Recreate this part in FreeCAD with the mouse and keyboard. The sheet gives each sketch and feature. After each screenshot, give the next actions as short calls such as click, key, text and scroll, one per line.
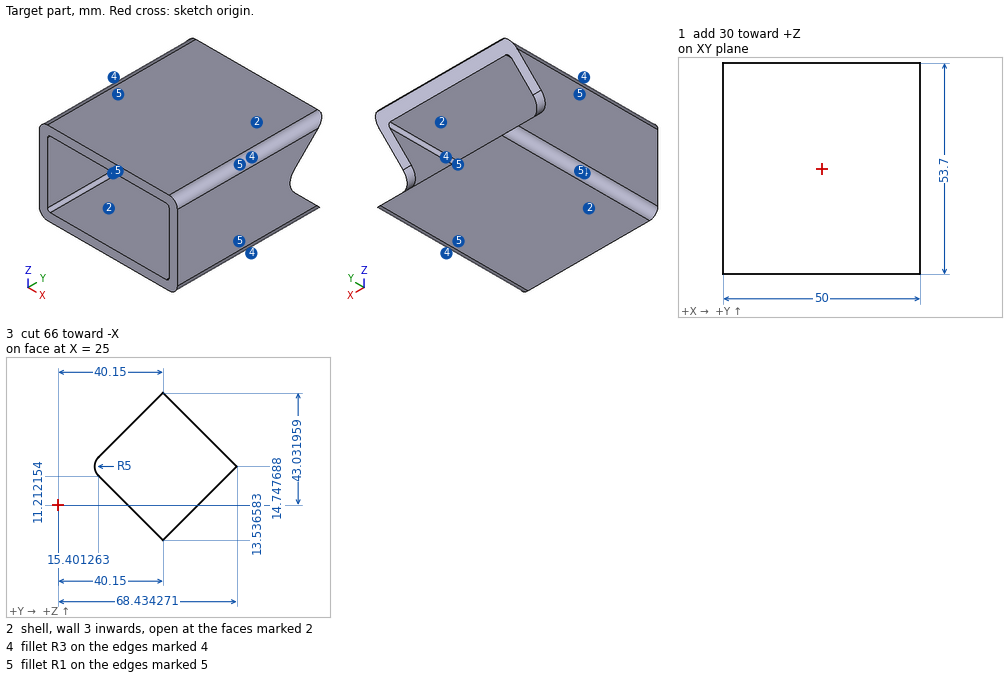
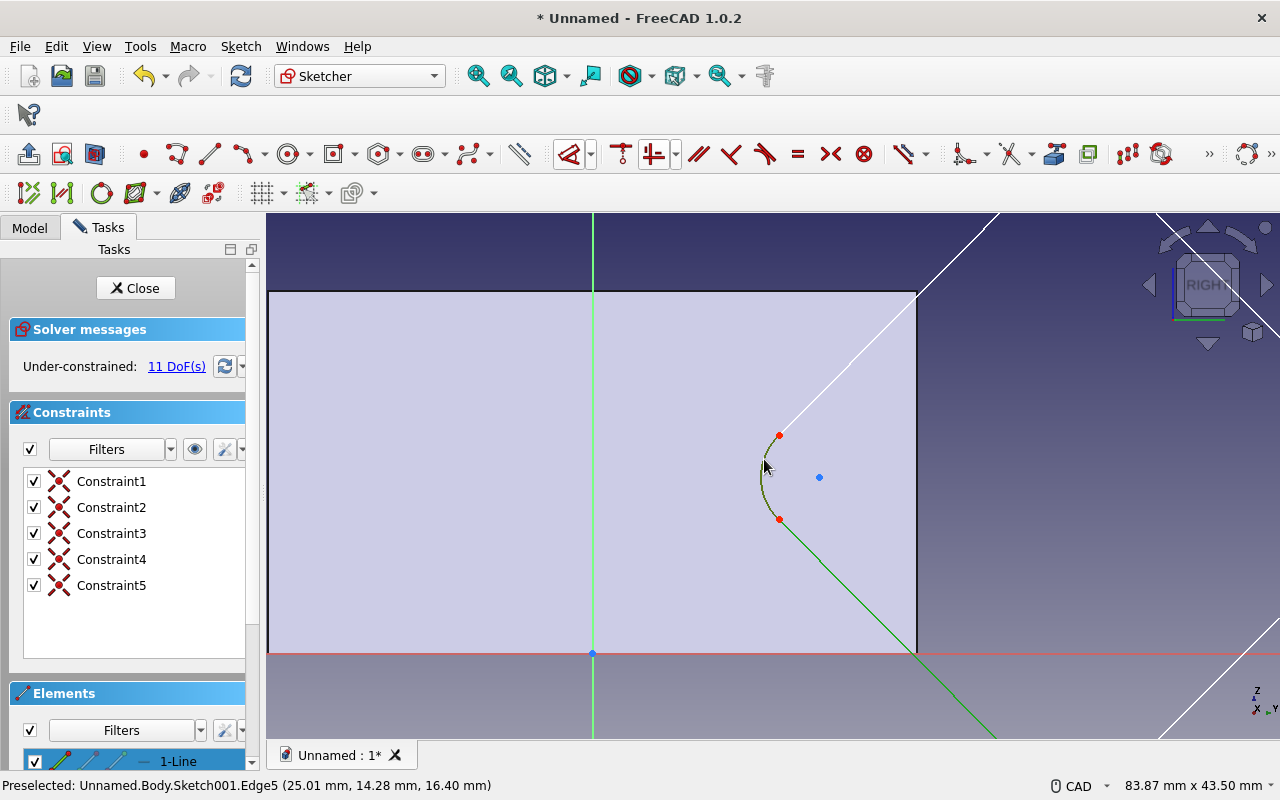
key(t)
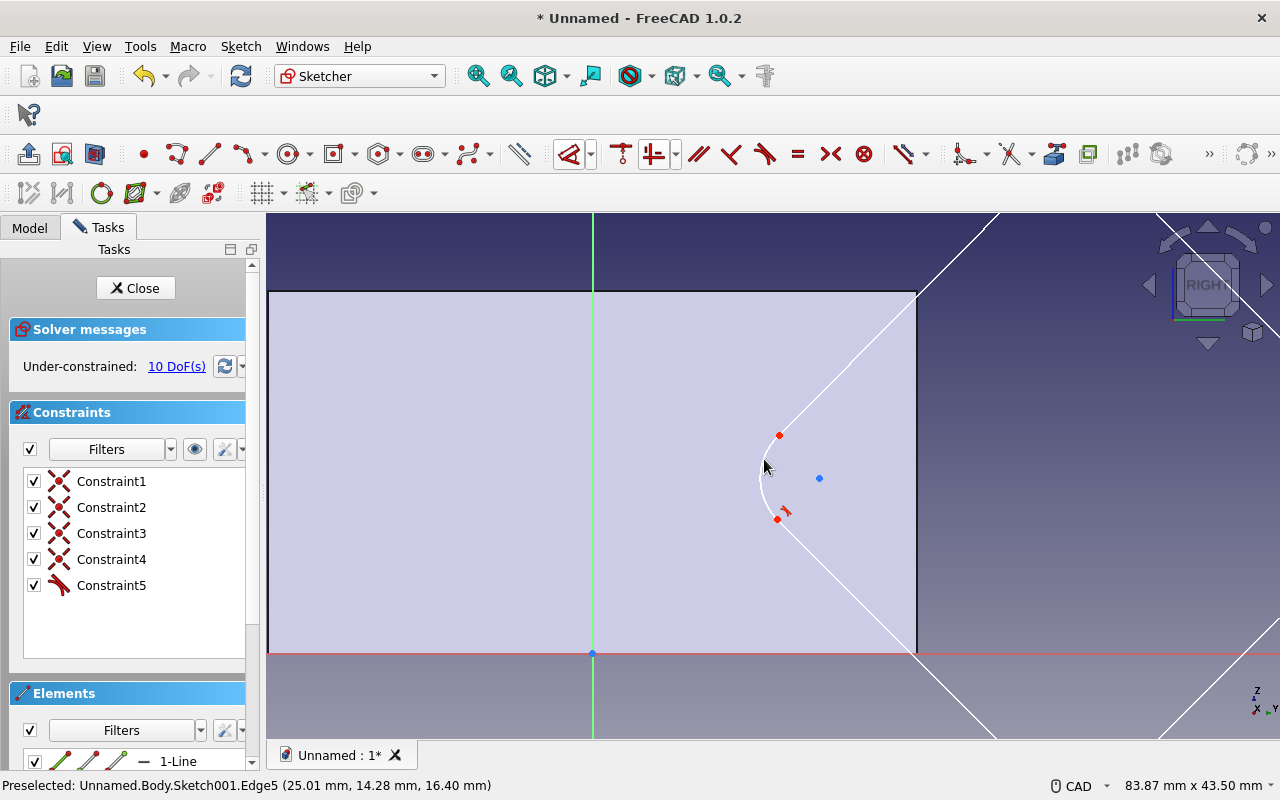
click(869, 345)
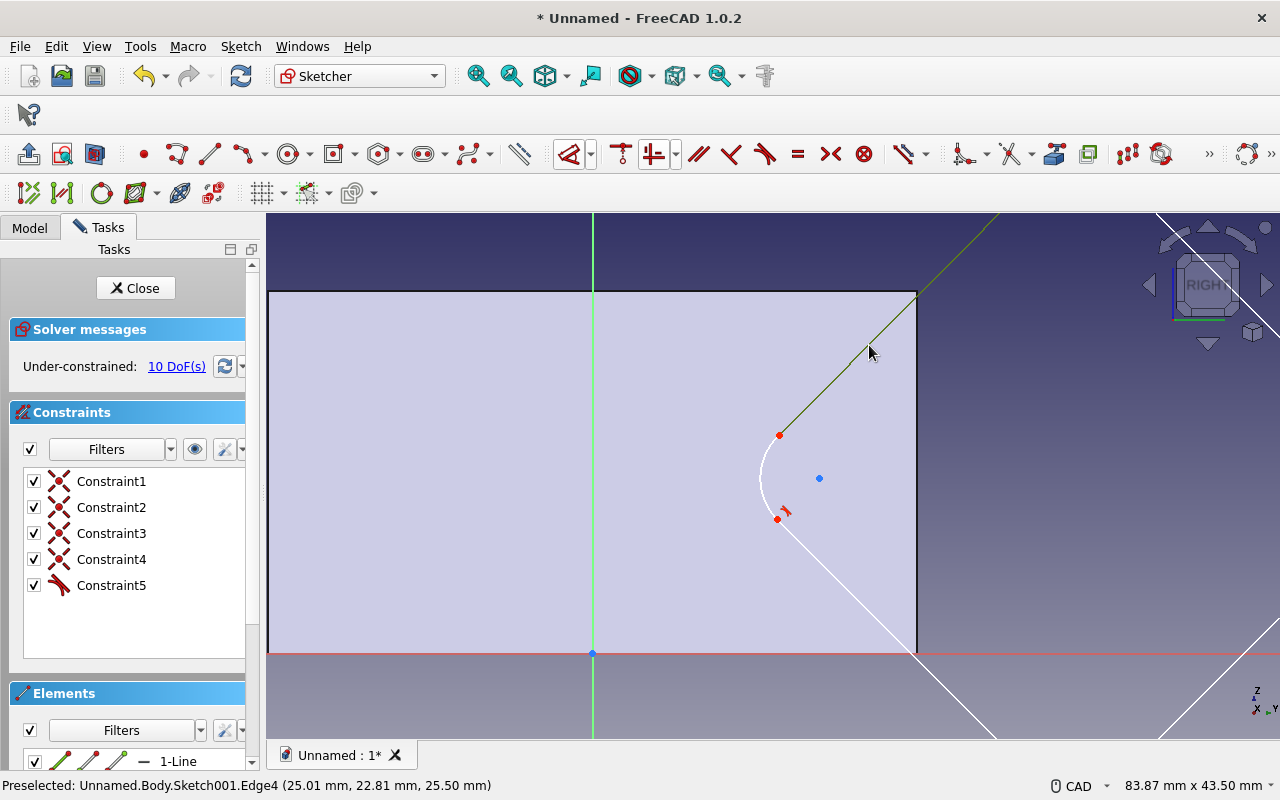
click(764, 459)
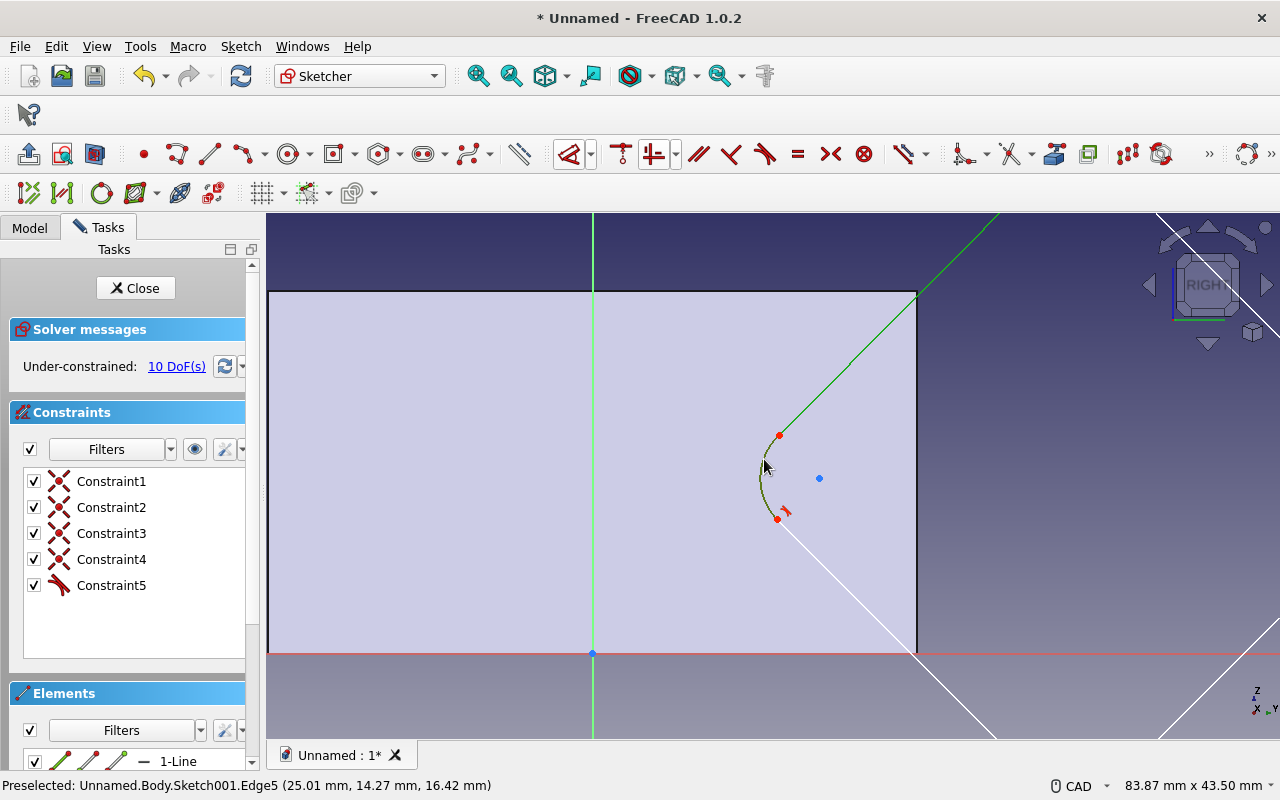
key(t)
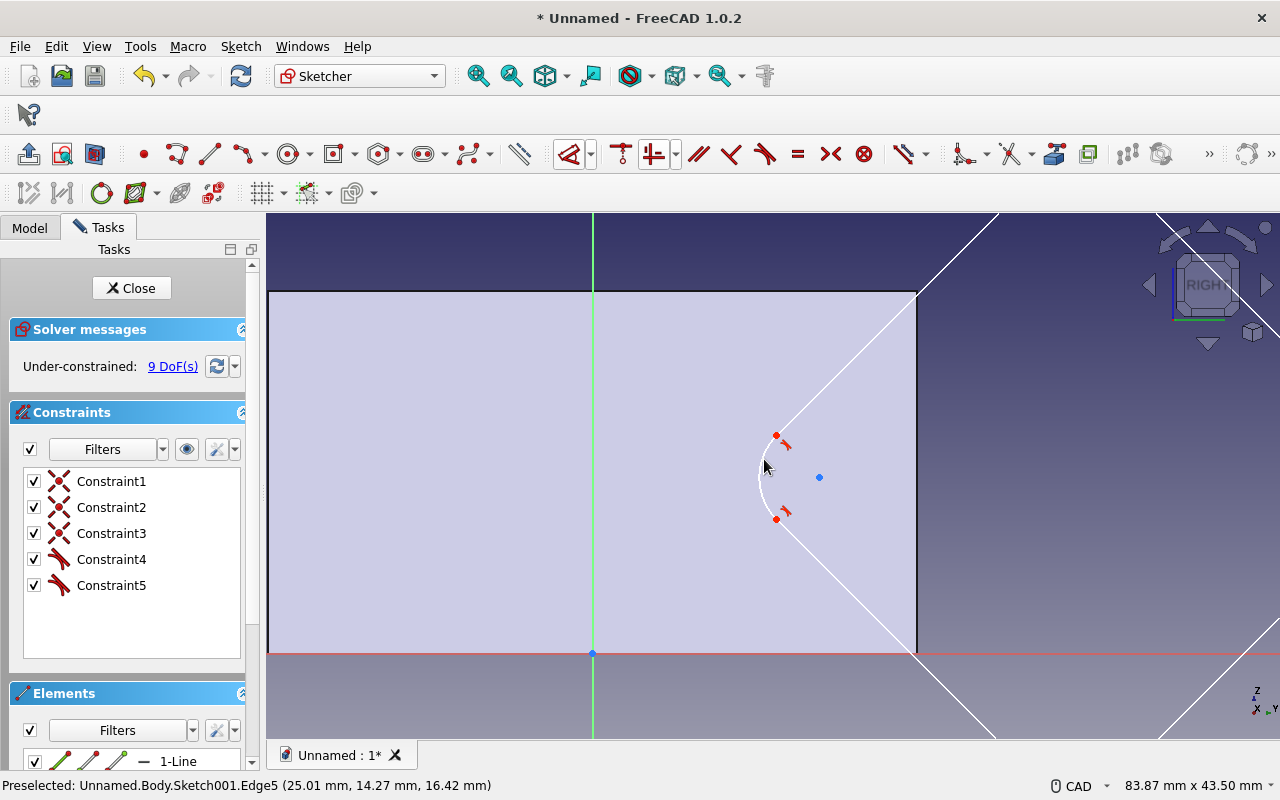
key(d)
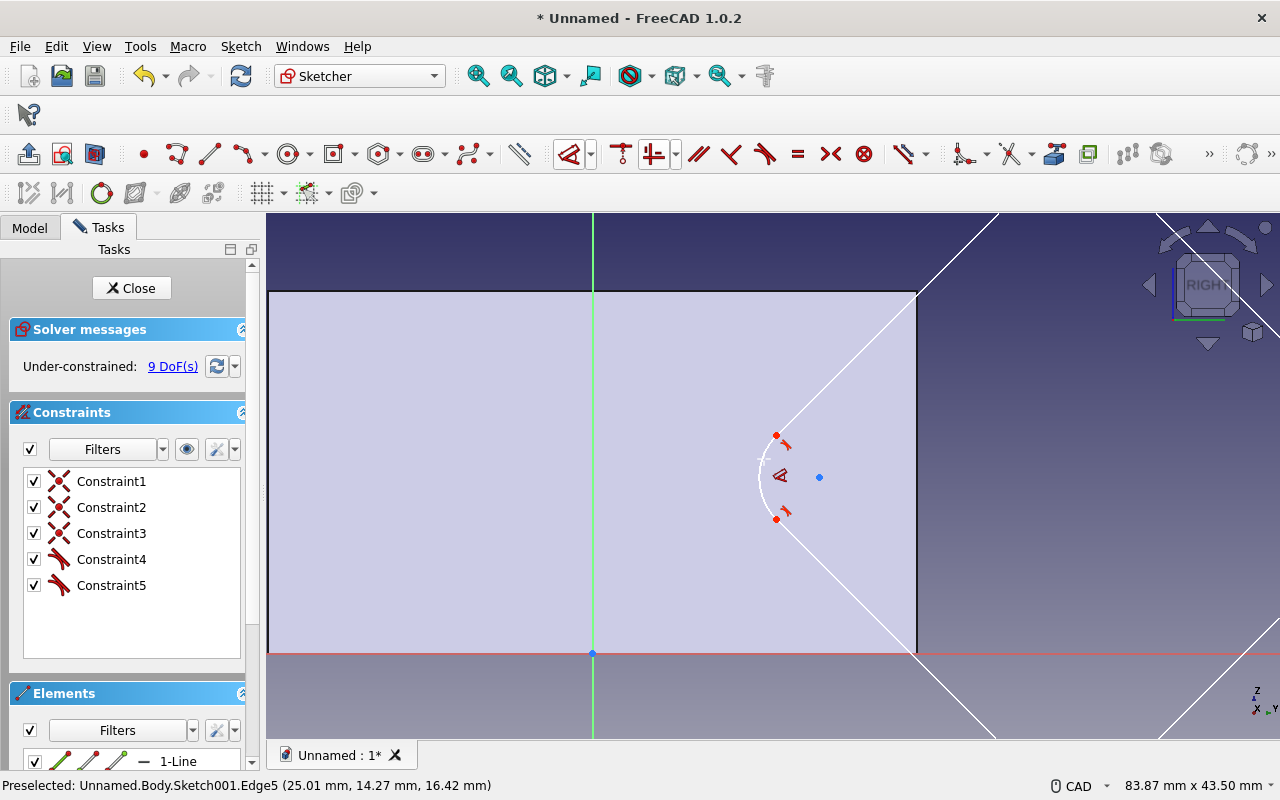
click(762, 459)
click(732, 449)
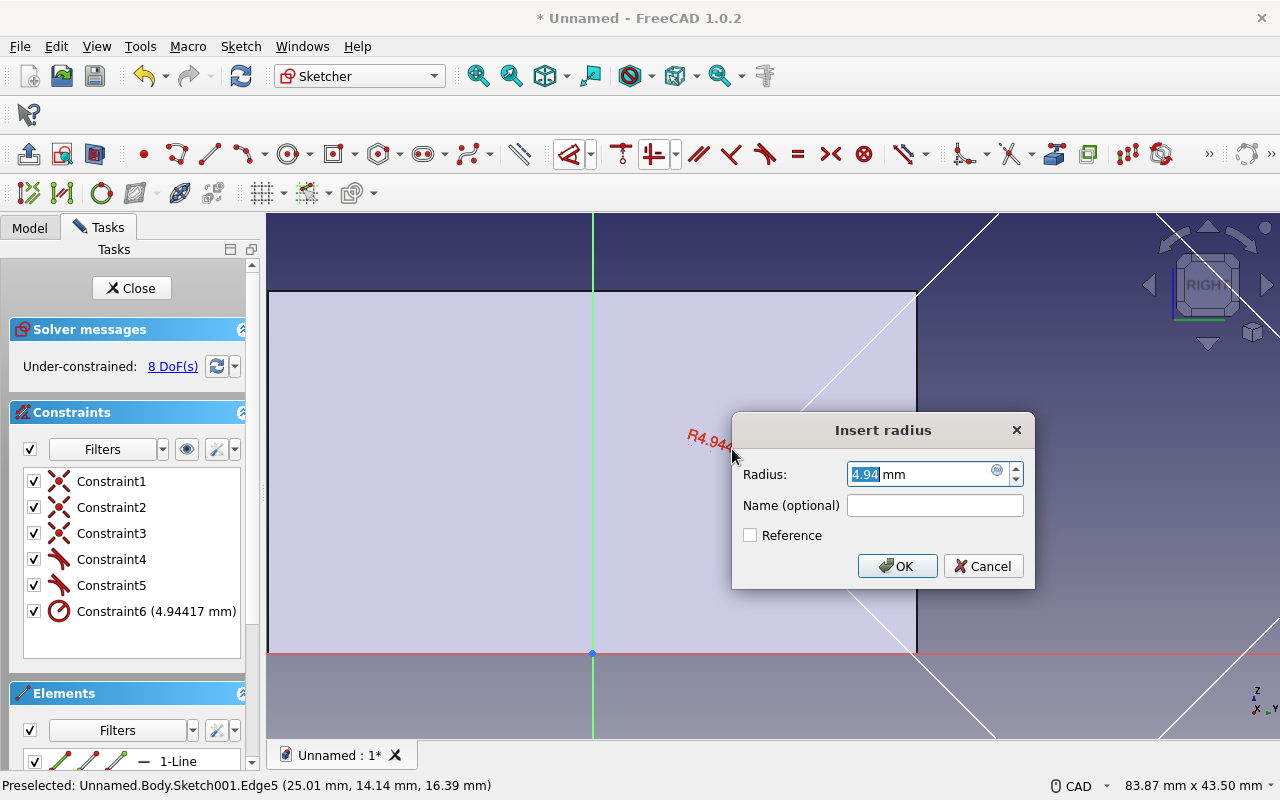
text(5)
key(Return)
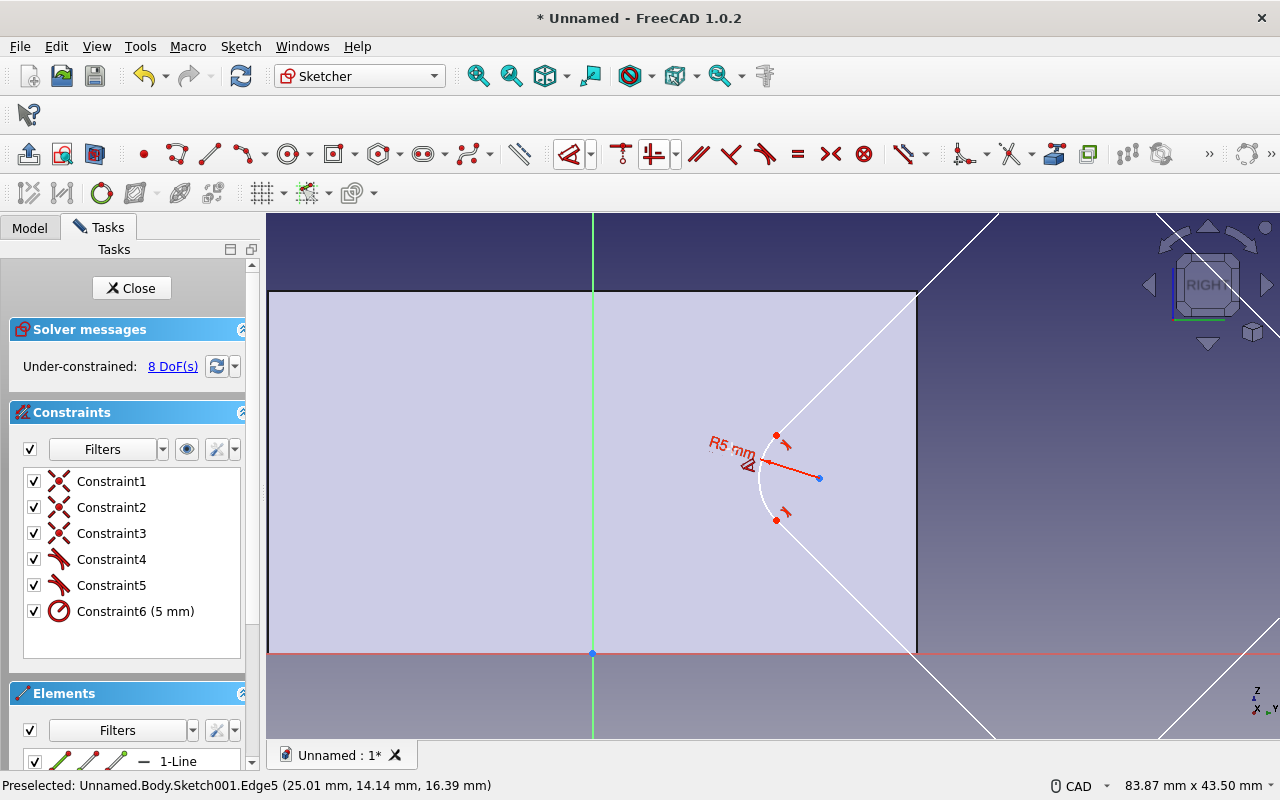
scroll(458, 476, down, 4)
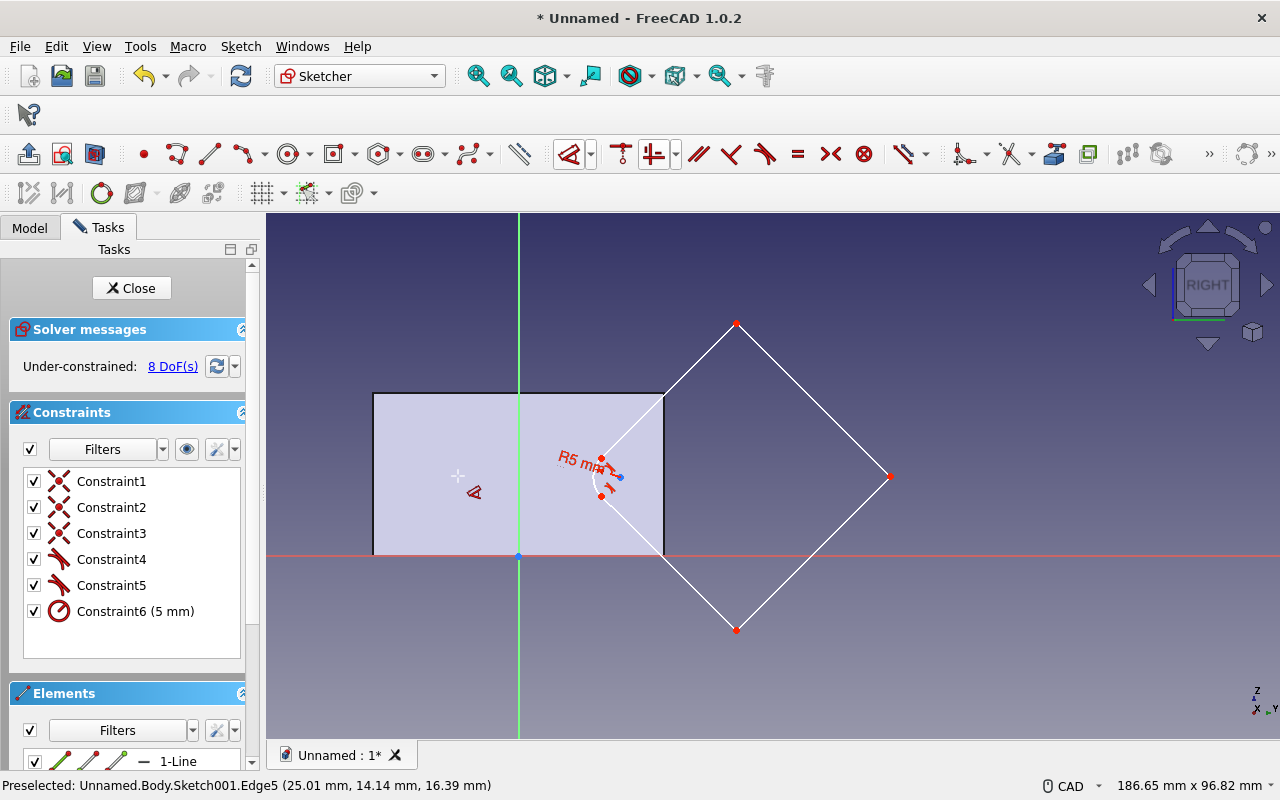
click(736, 631)
click(628, 665)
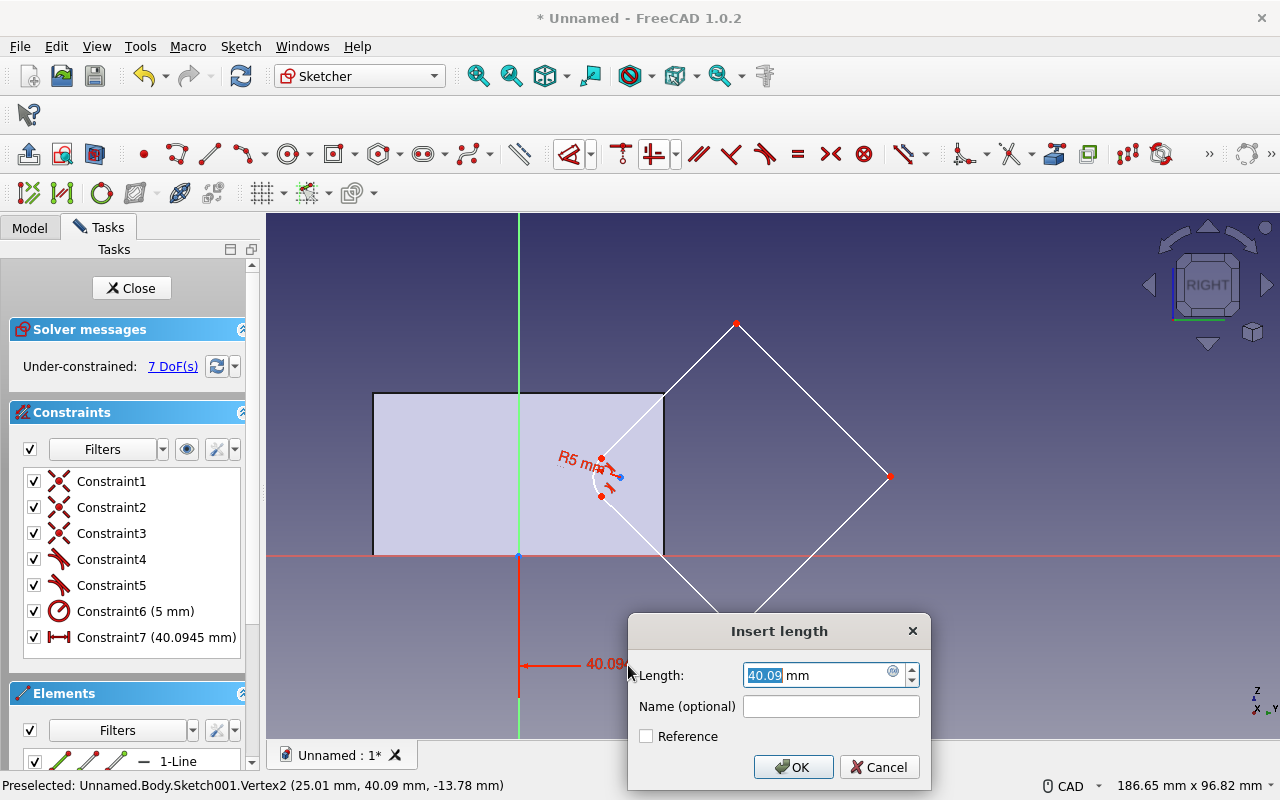
text(40.15)
key(Return)